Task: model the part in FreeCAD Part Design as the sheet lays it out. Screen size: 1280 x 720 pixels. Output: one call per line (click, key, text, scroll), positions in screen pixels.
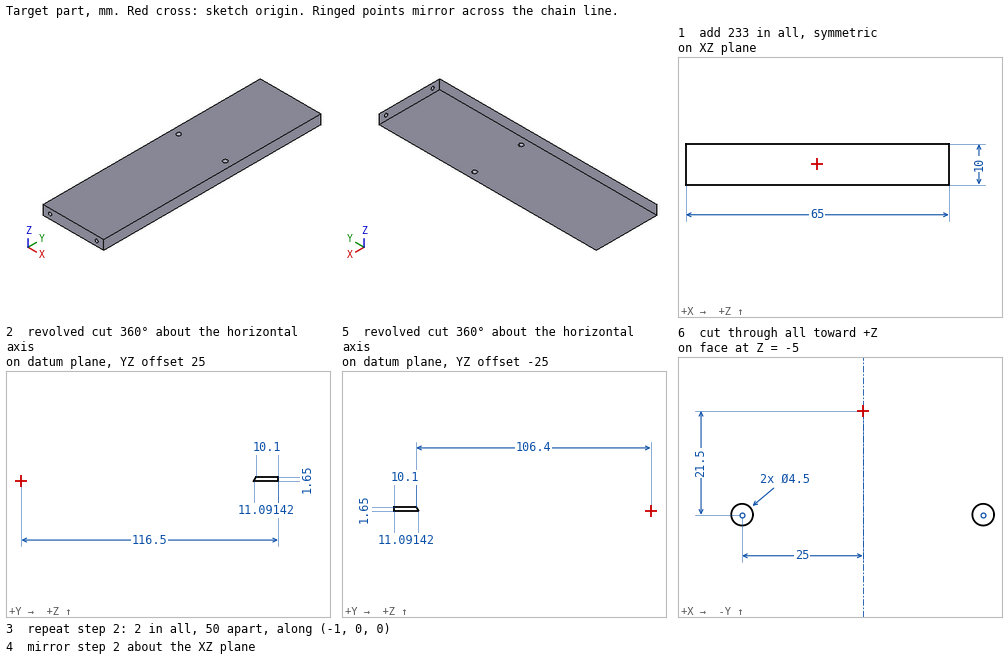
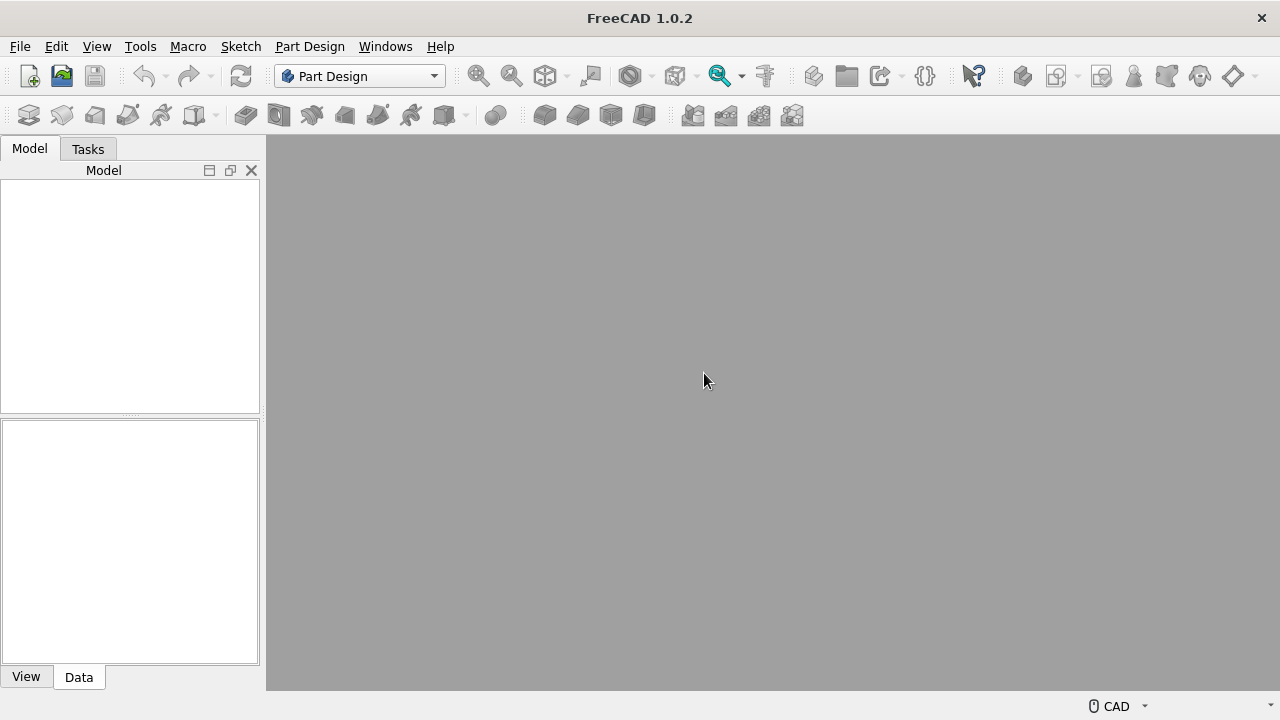
key(ctrl+n)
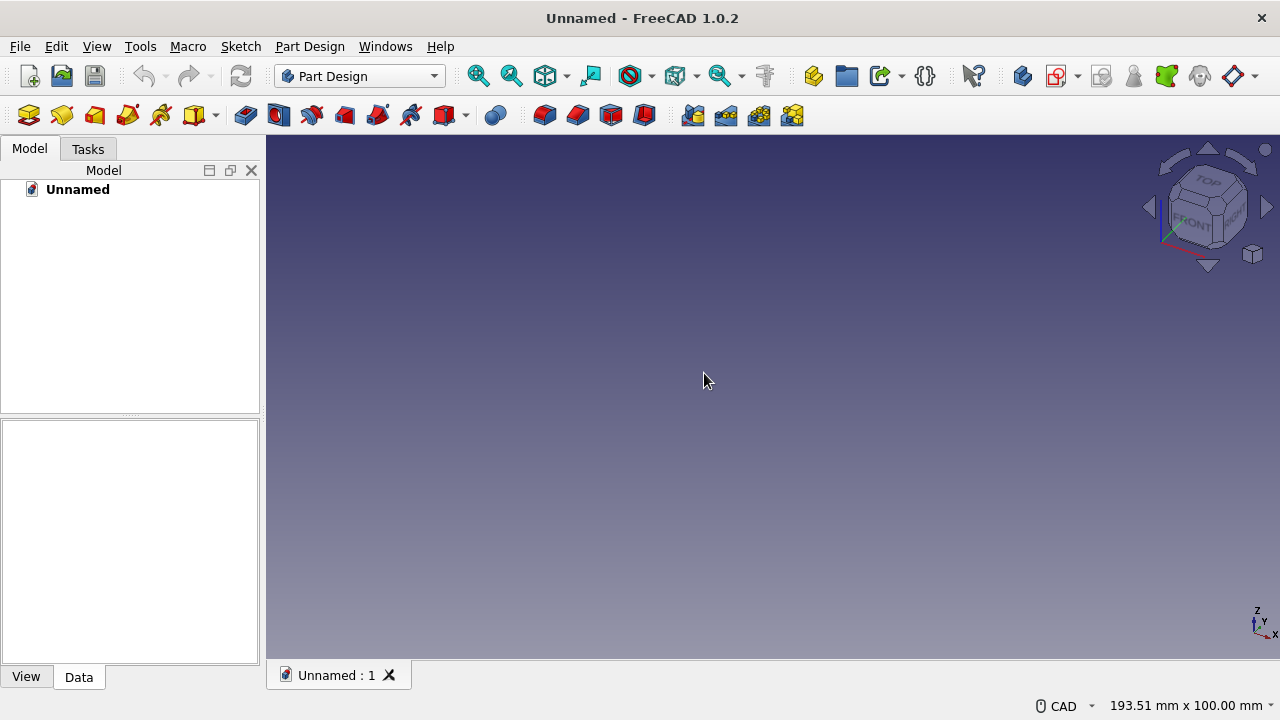
click(1056, 76)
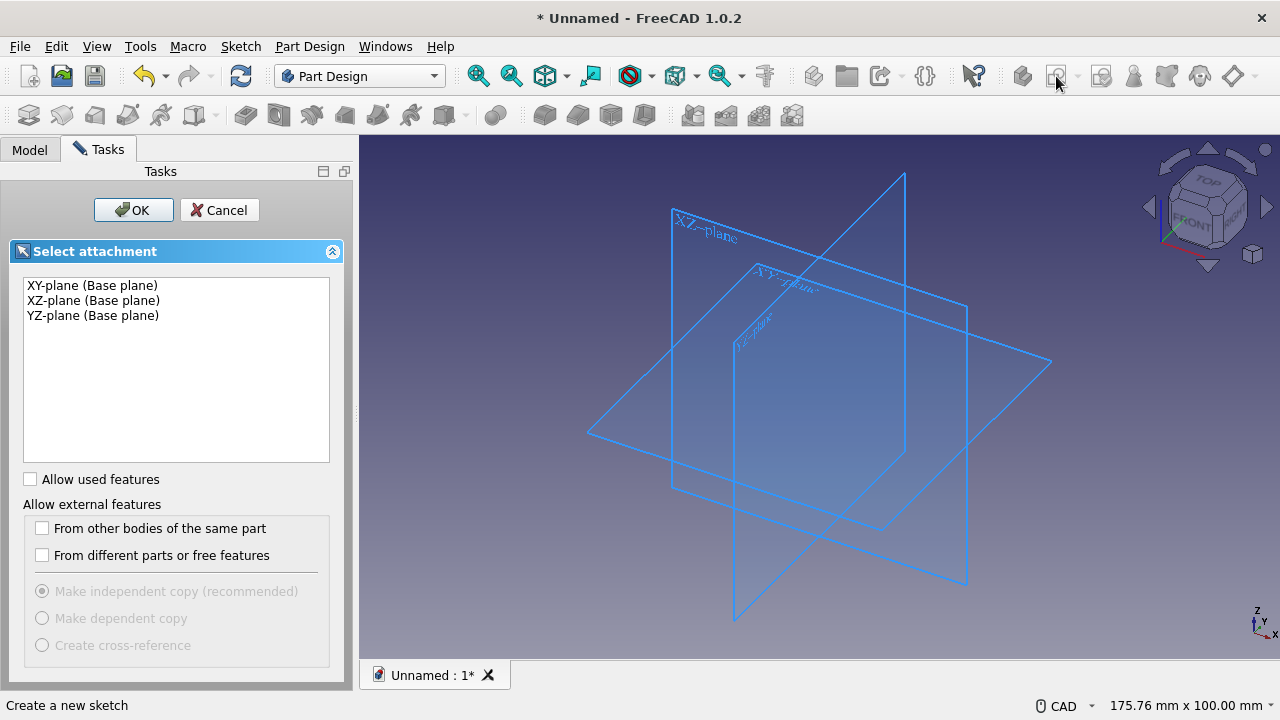
click(84, 300)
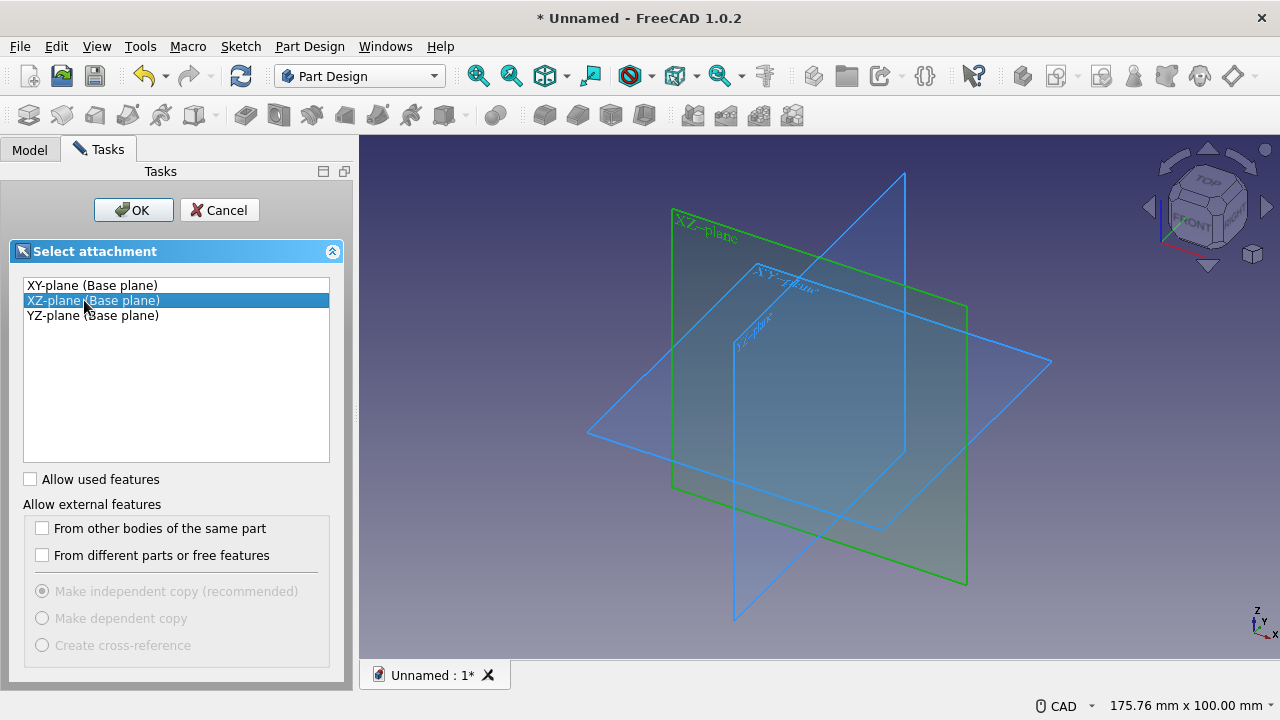
click(134, 210)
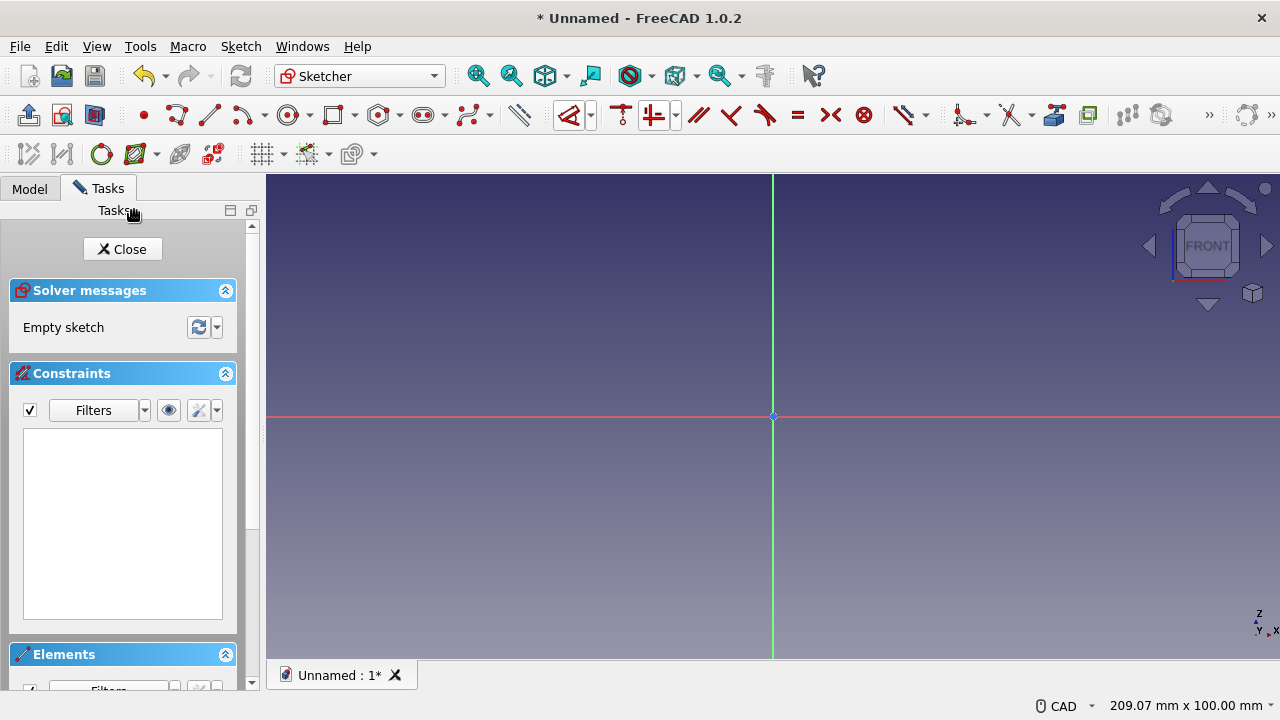
scroll(856, 416, up, 3)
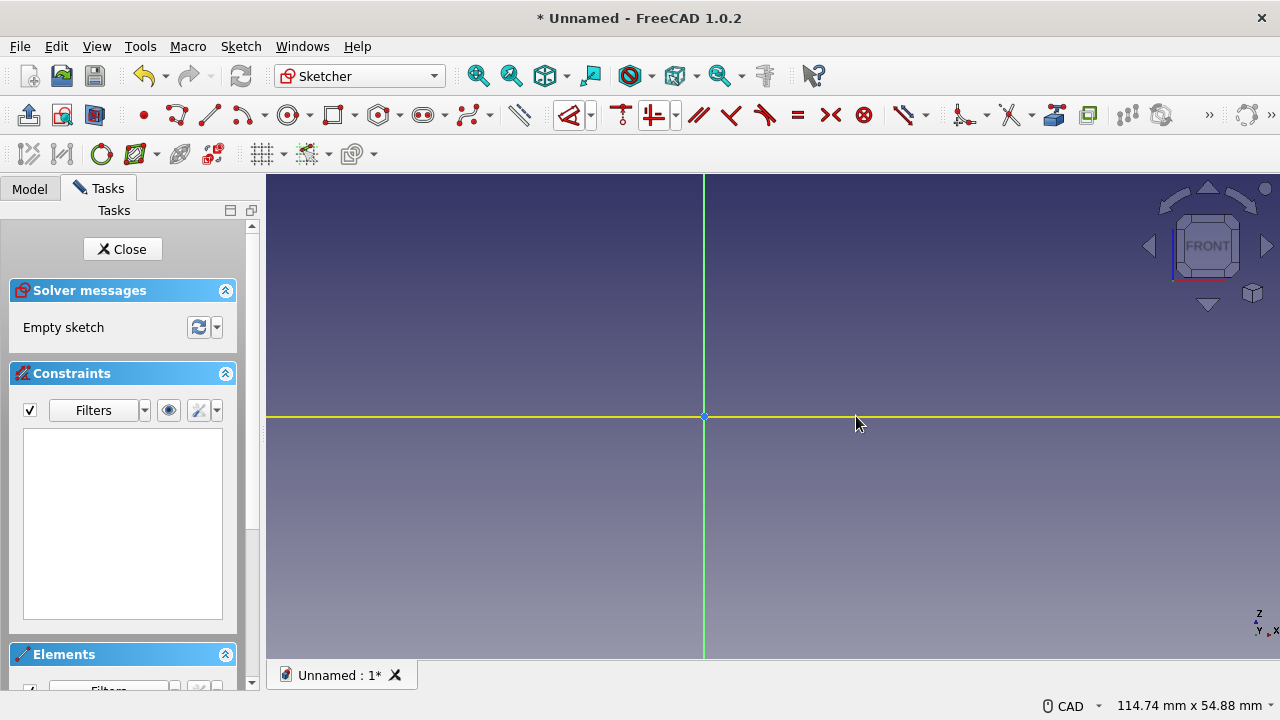
key(g)
key(v)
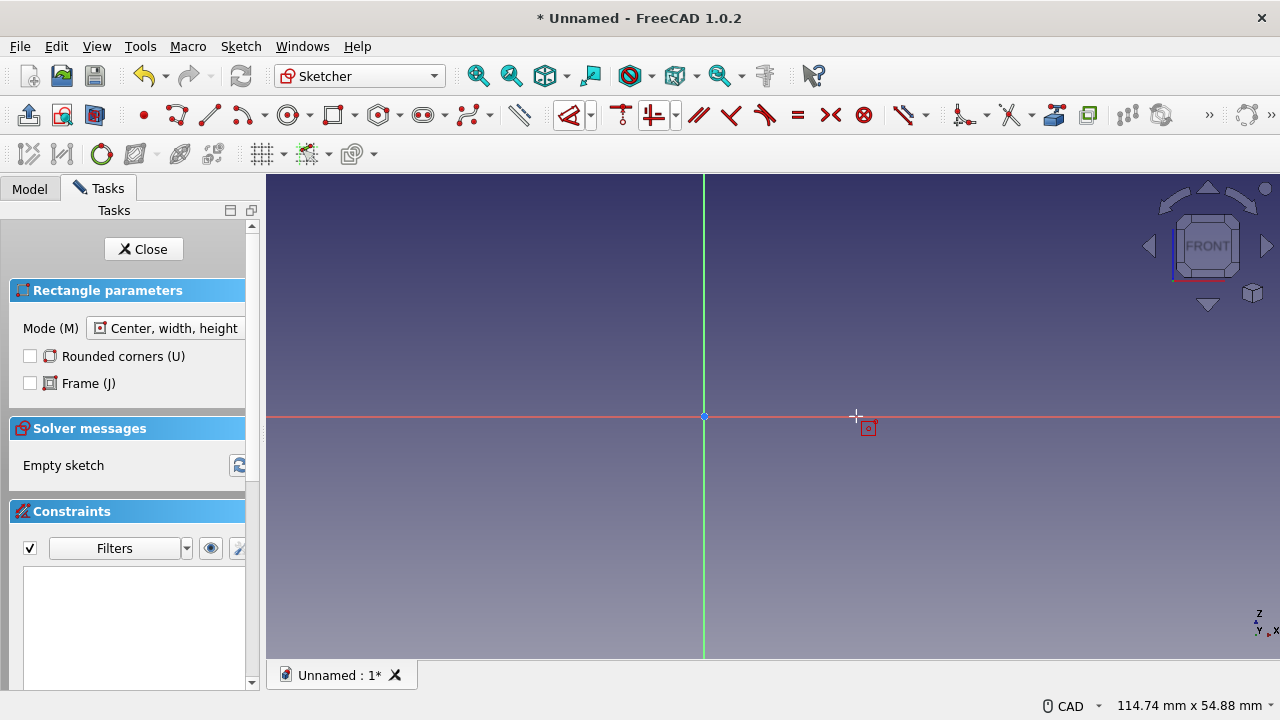
click(704, 416)
click(991, 372)
key(Escape)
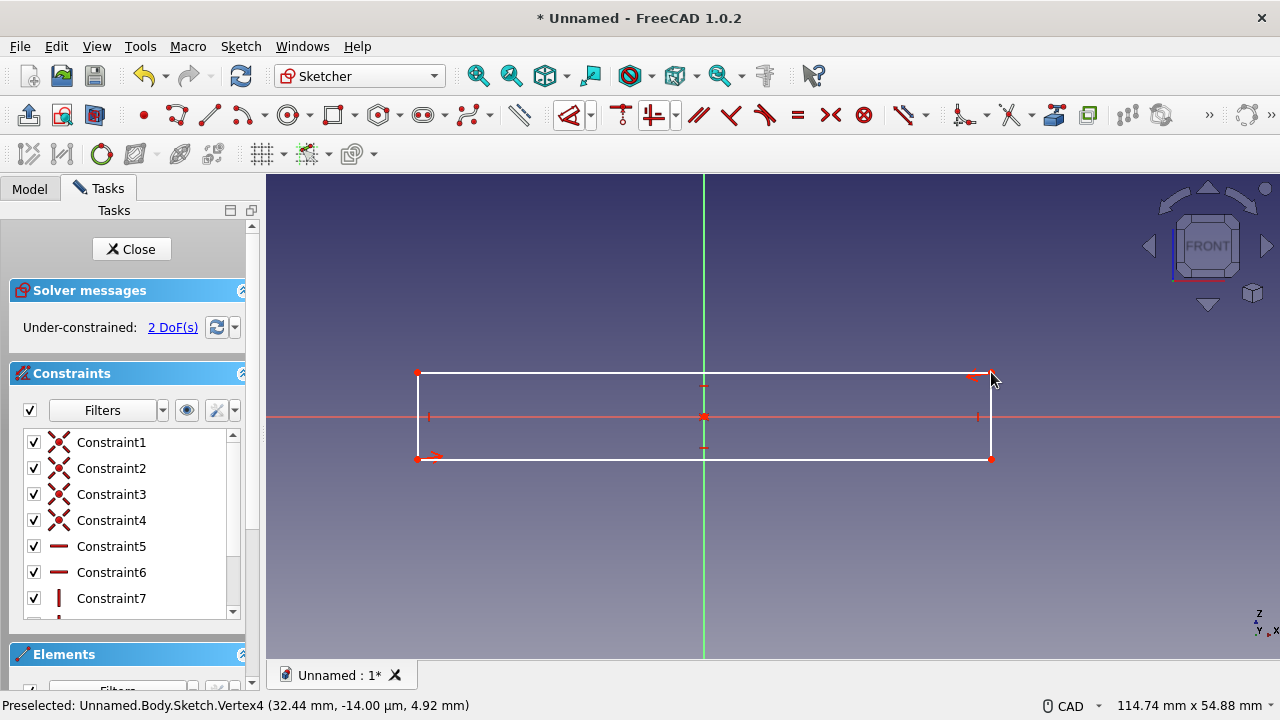
key(d)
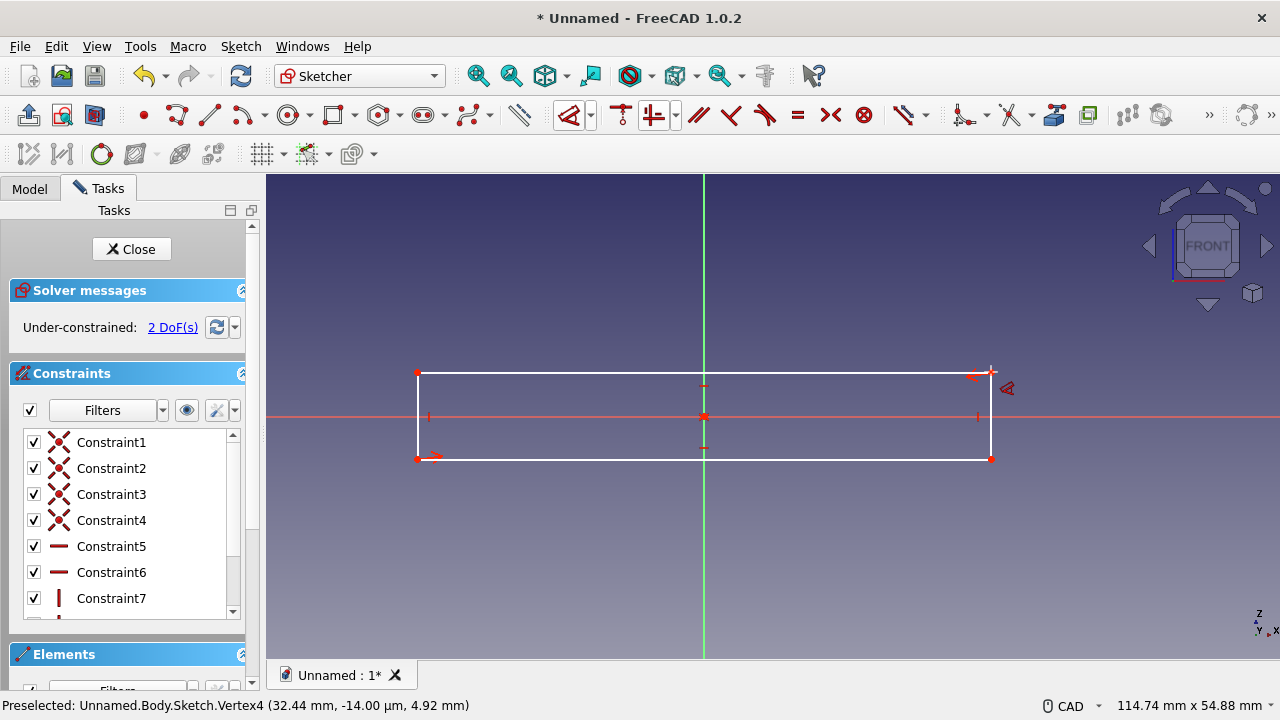
click(590, 460)
click(572, 494)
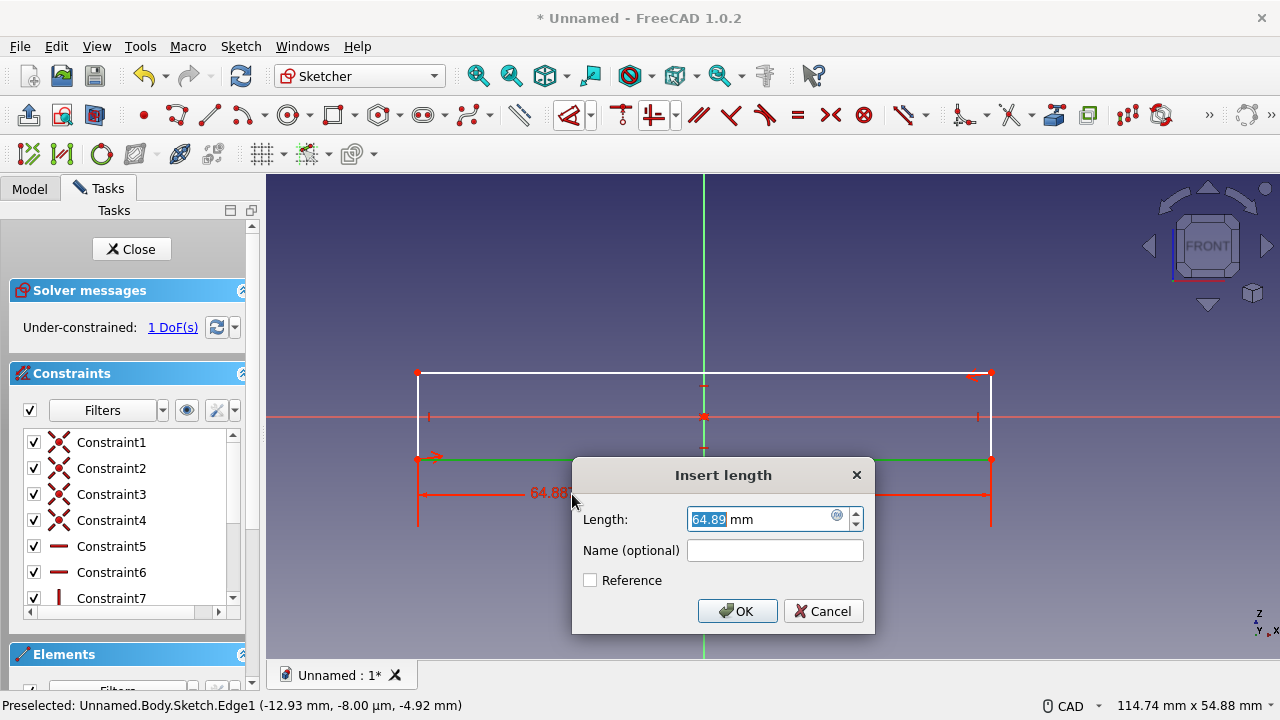
text(65)
key(Return)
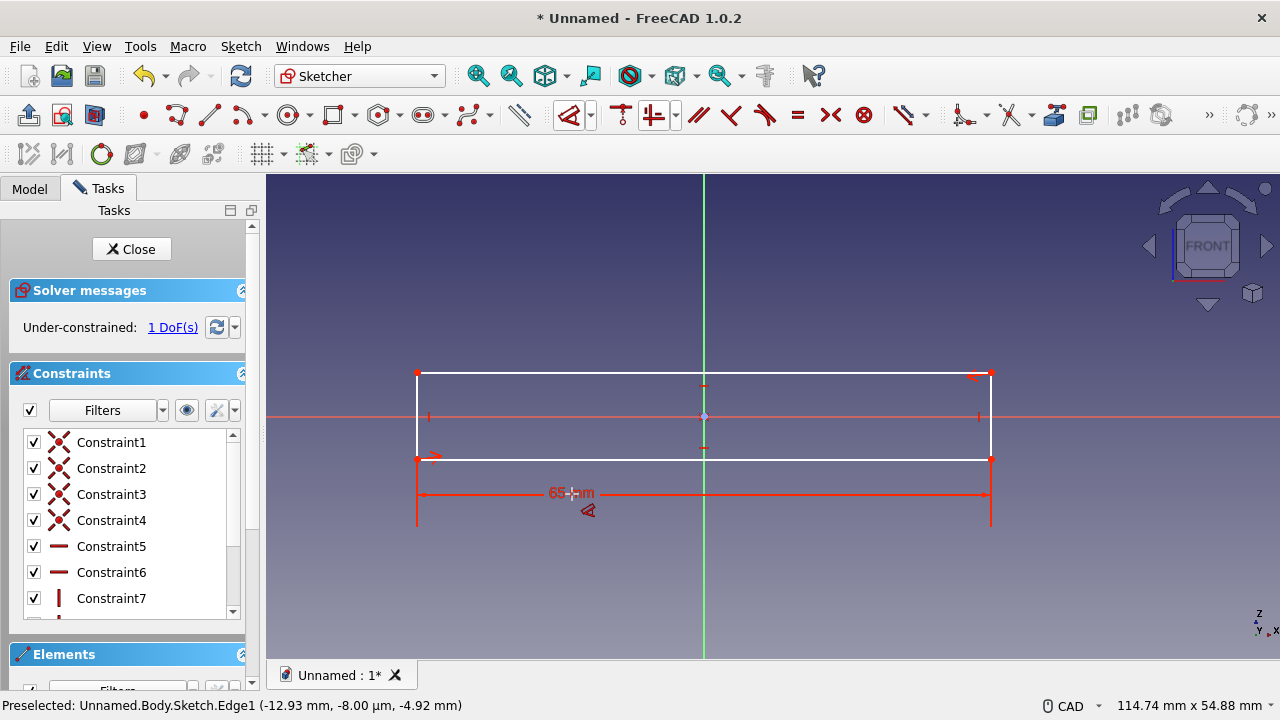
click(991, 434)
click(1025, 396)